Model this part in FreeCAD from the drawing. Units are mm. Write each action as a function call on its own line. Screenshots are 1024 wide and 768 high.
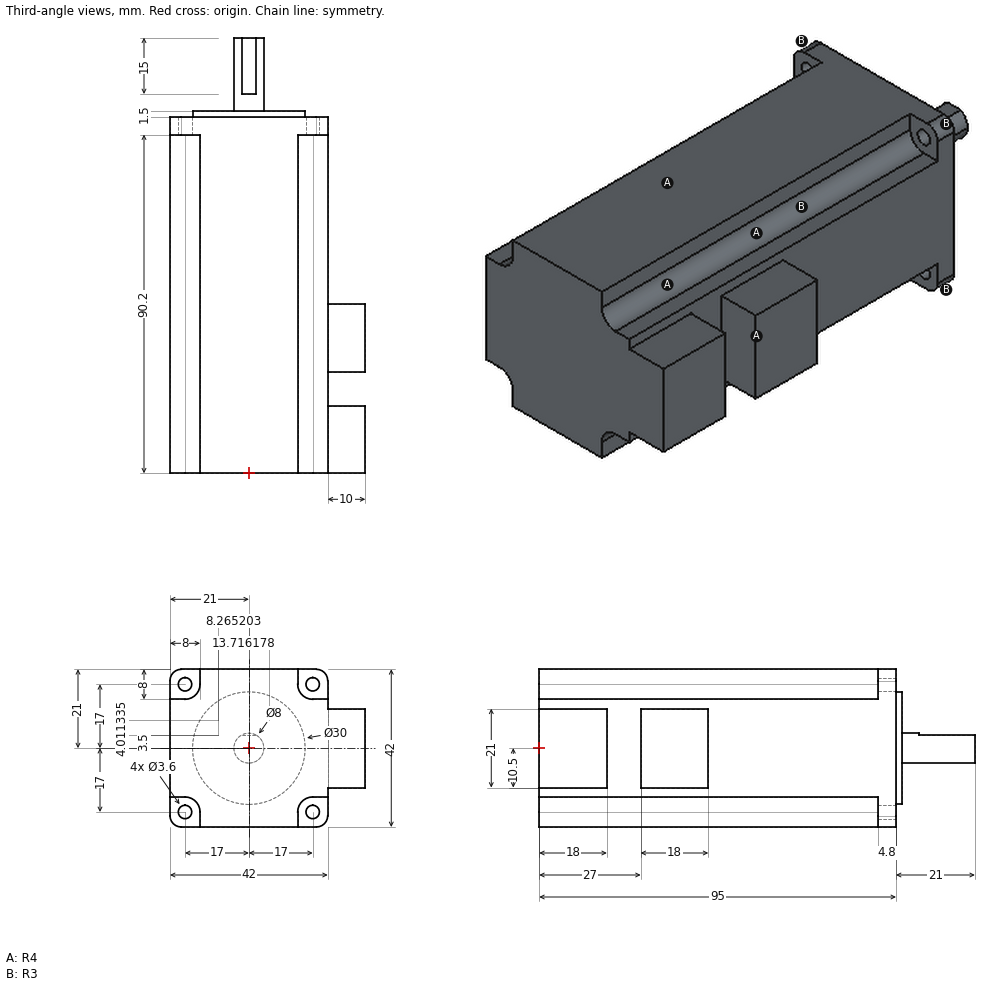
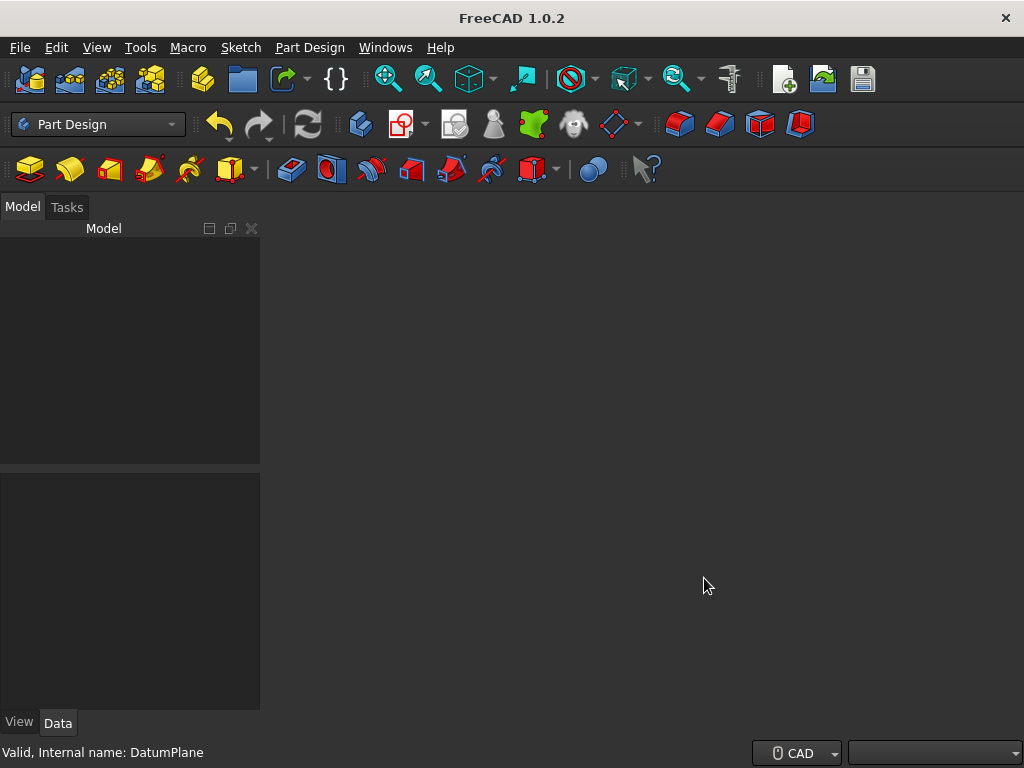
key(ctrl+n)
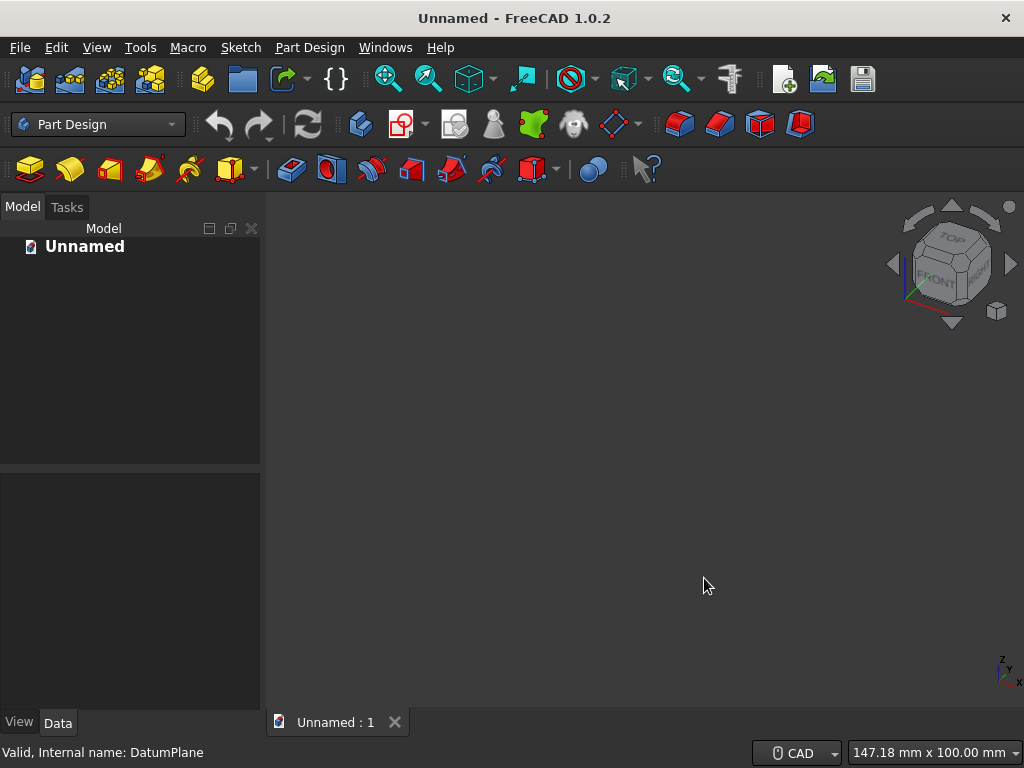
click(402, 124)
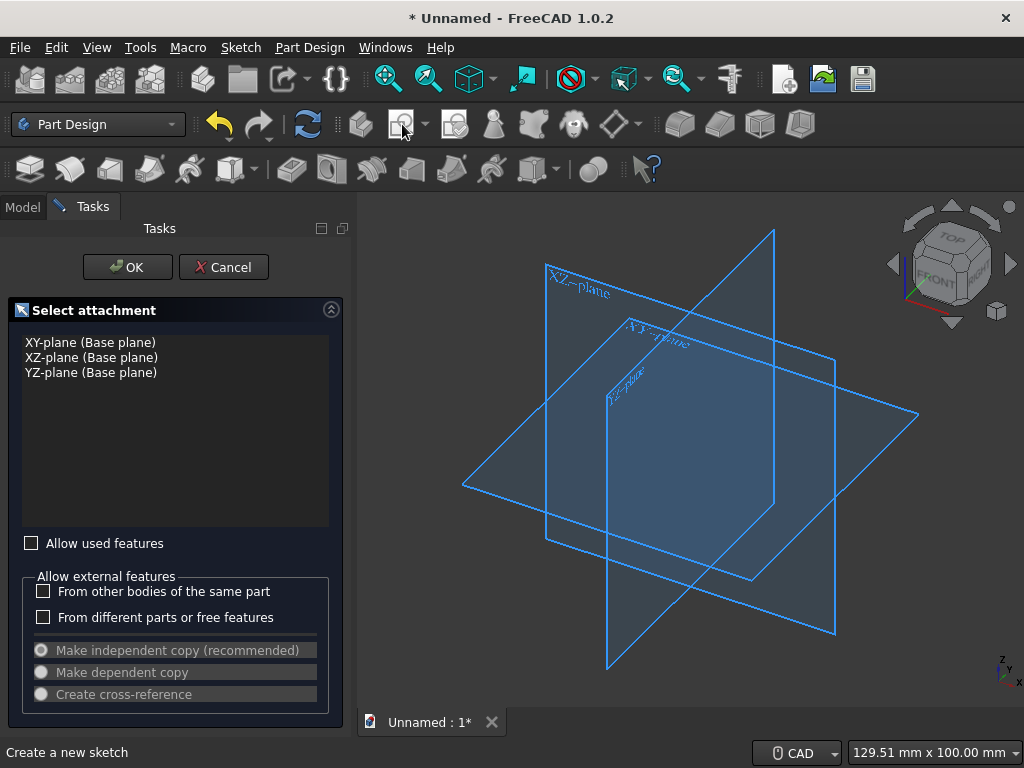
click(82, 358)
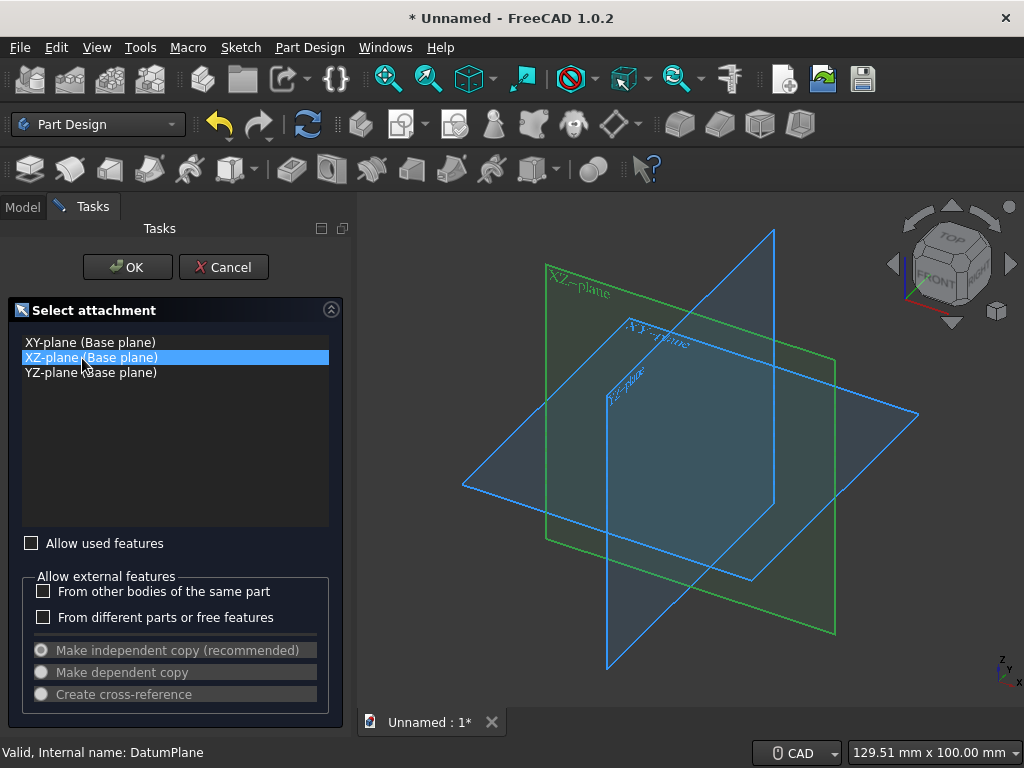
click(128, 267)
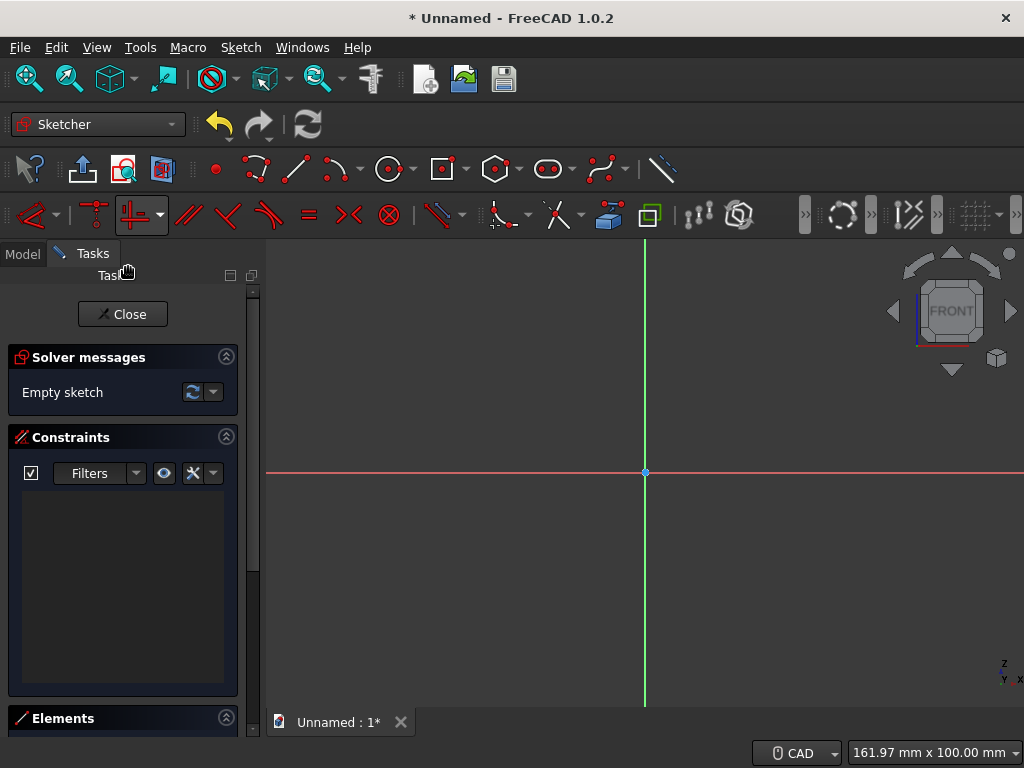
scroll(784, 473, up, 2)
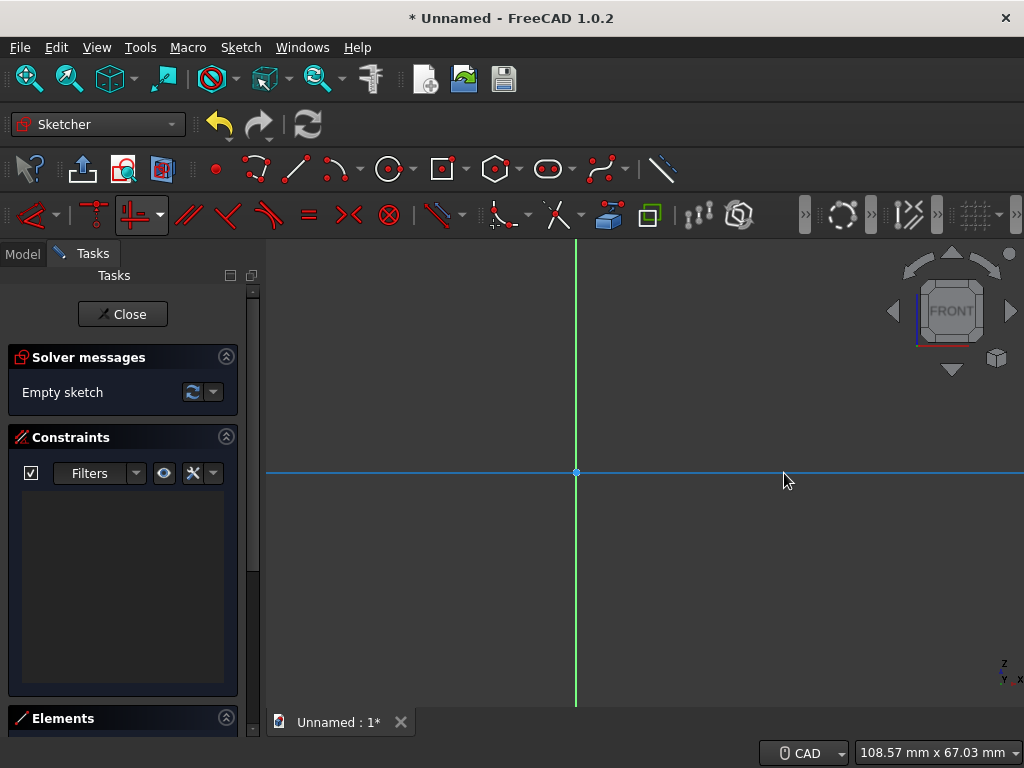
key(g)
key(v)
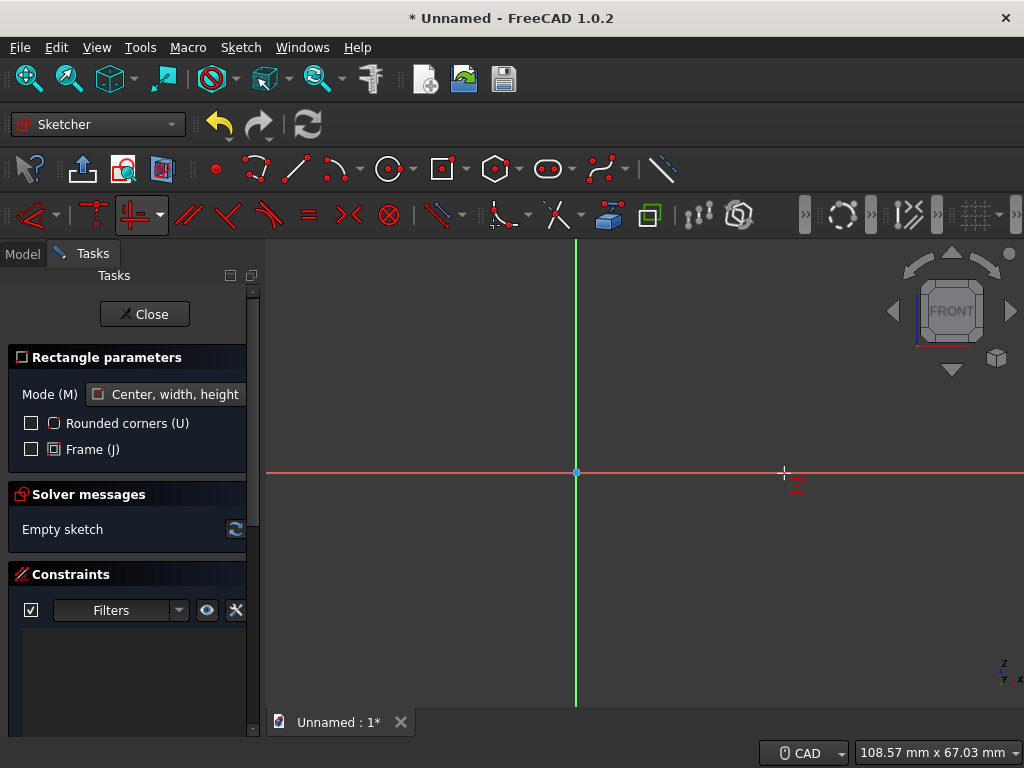
click(576, 473)
click(723, 326)
key(Escape)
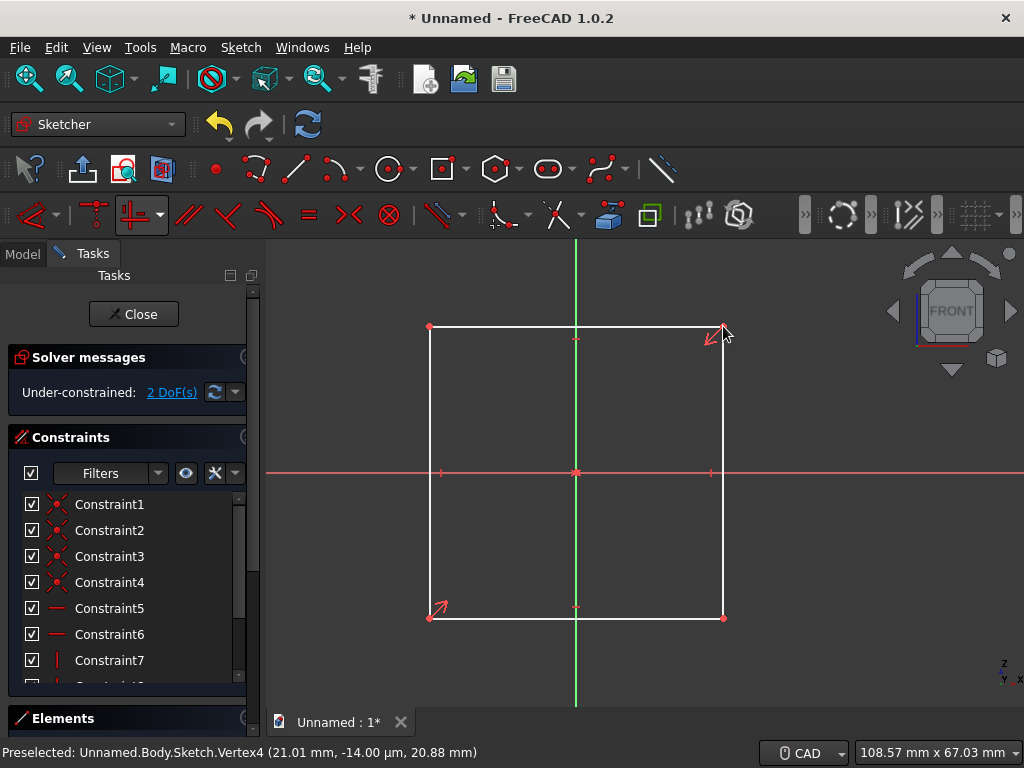
click(32, 216)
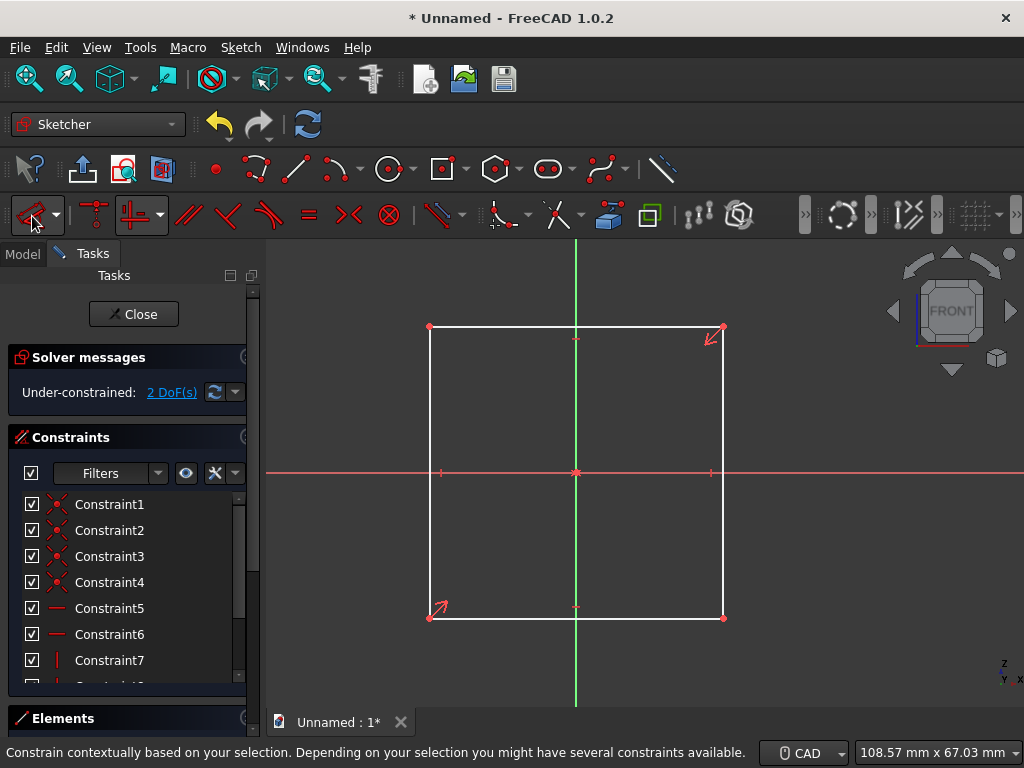
click(518, 619)
click(509, 653)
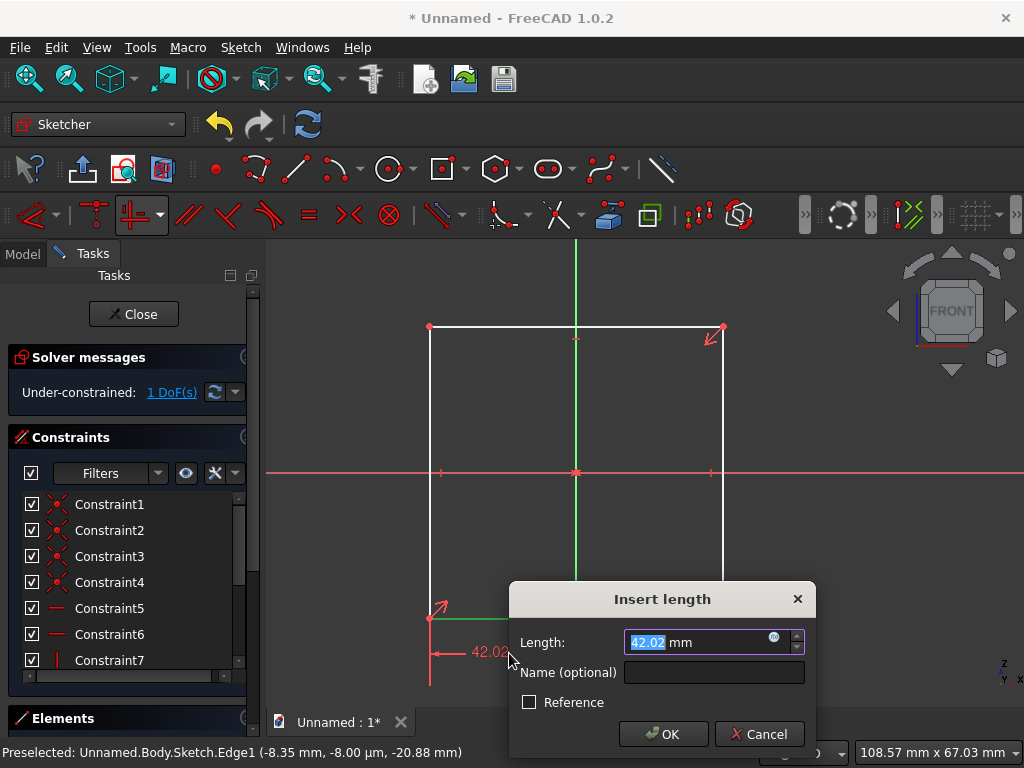
text(42)
key(Return)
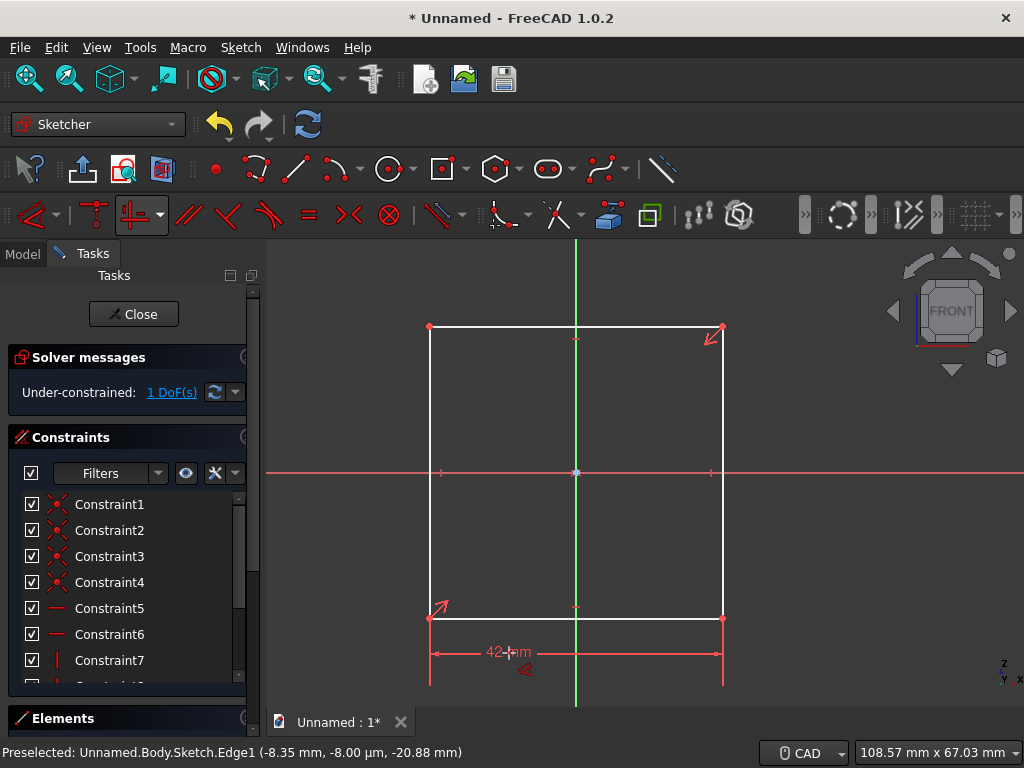
click(723, 531)
click(757, 406)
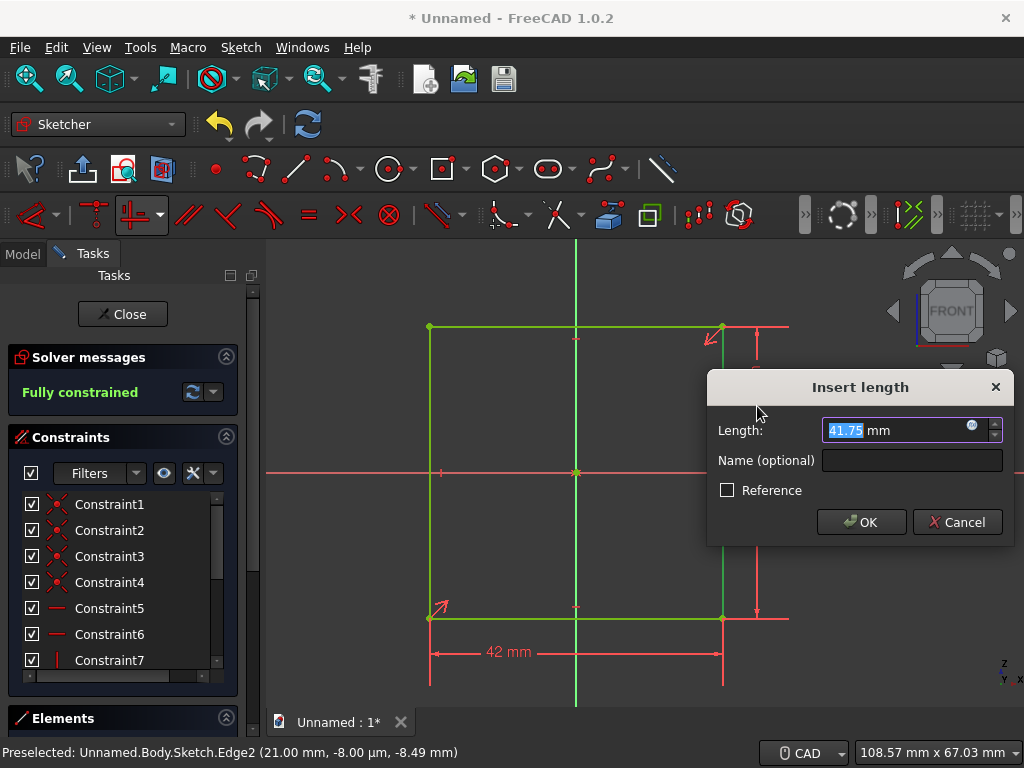
text(42)
key(Return)
key(Escape)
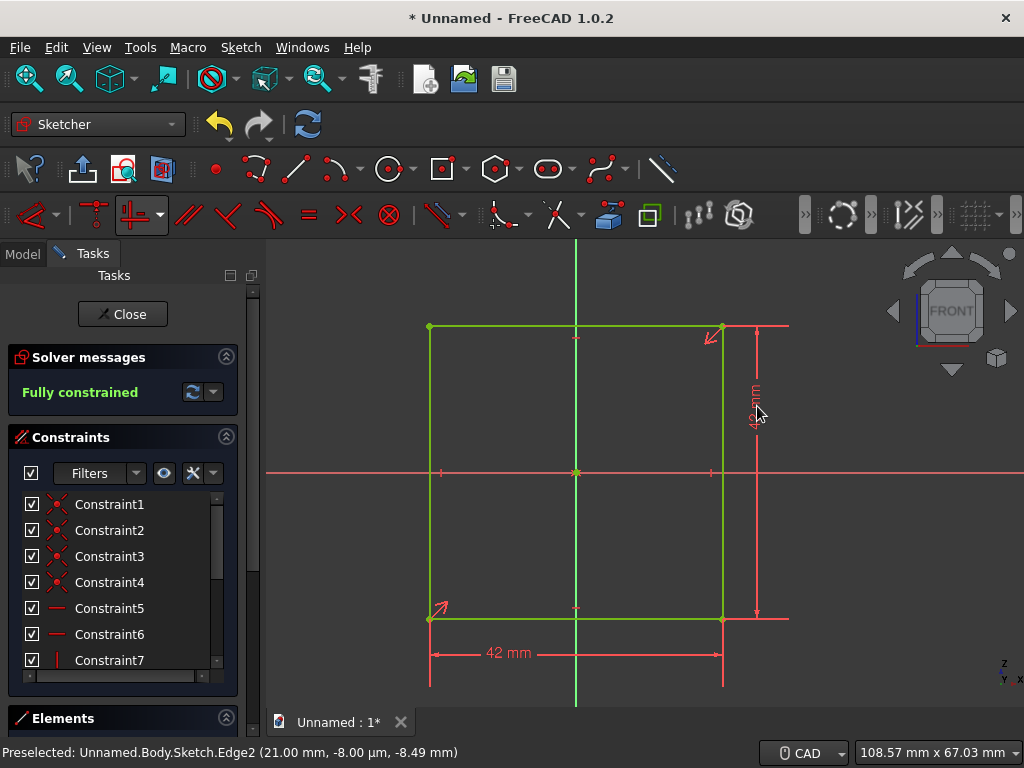
click(123, 314)